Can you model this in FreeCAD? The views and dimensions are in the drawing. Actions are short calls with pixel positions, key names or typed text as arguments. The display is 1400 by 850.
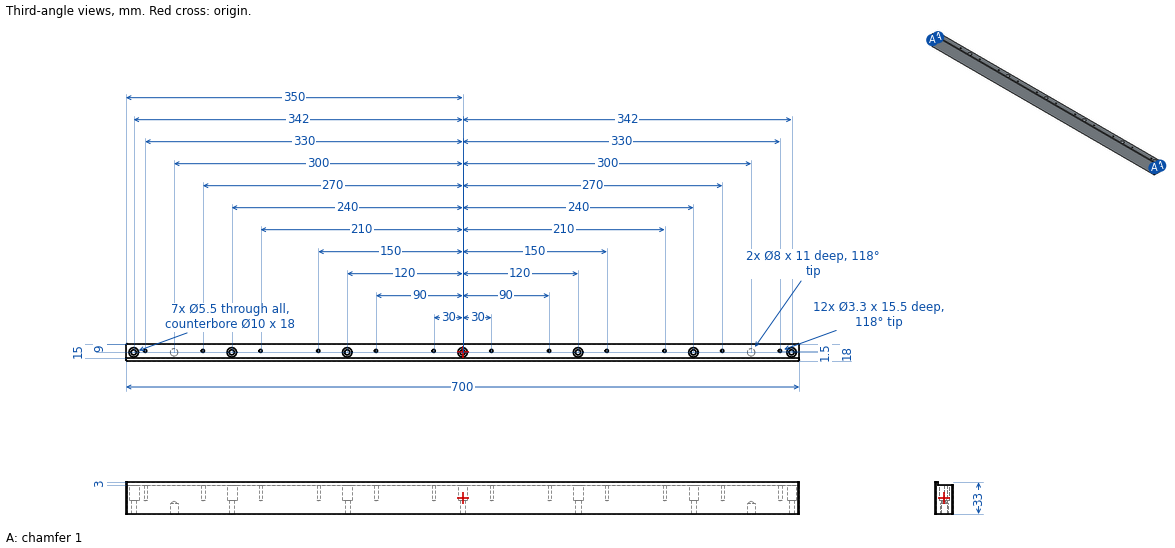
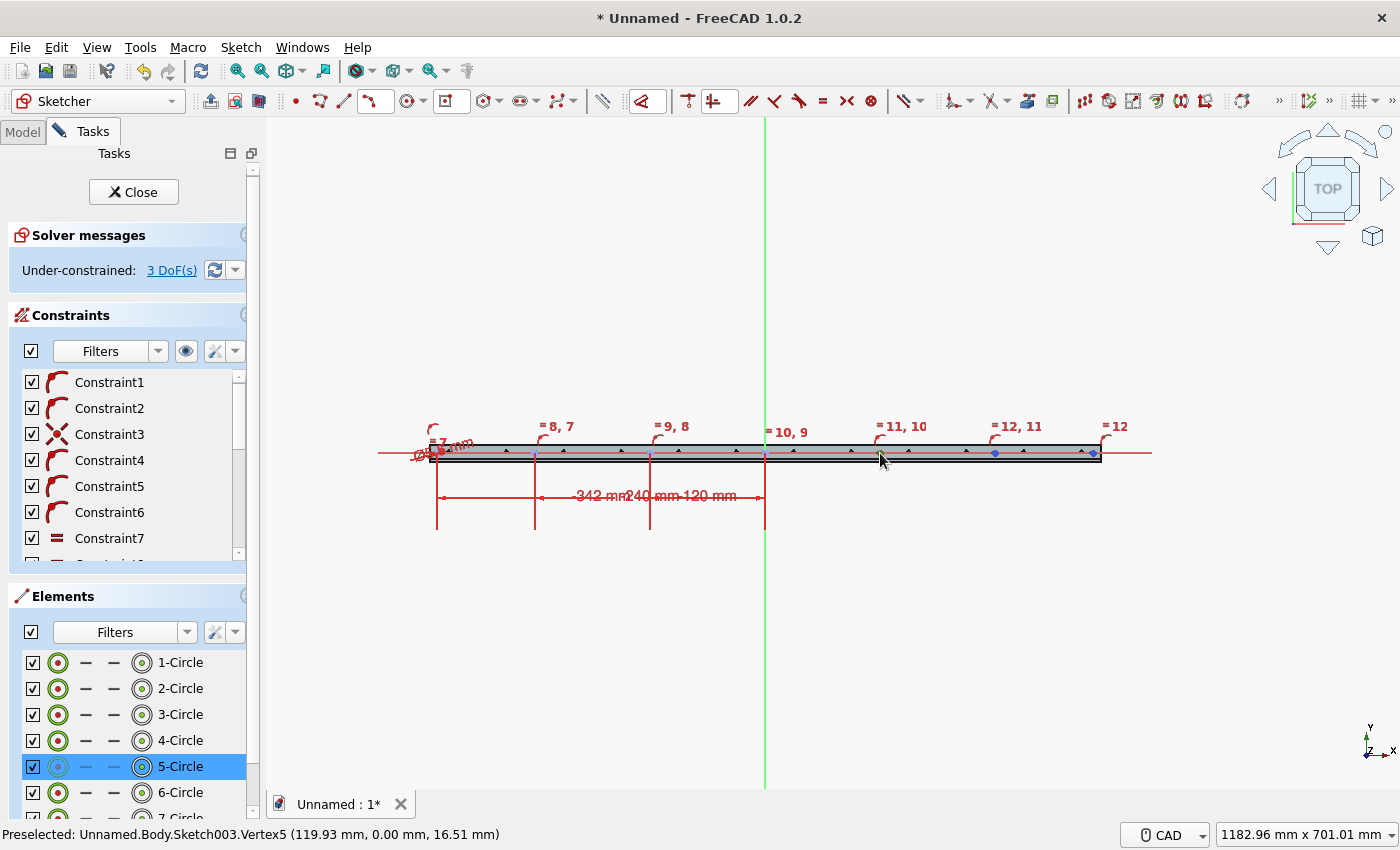
key(l)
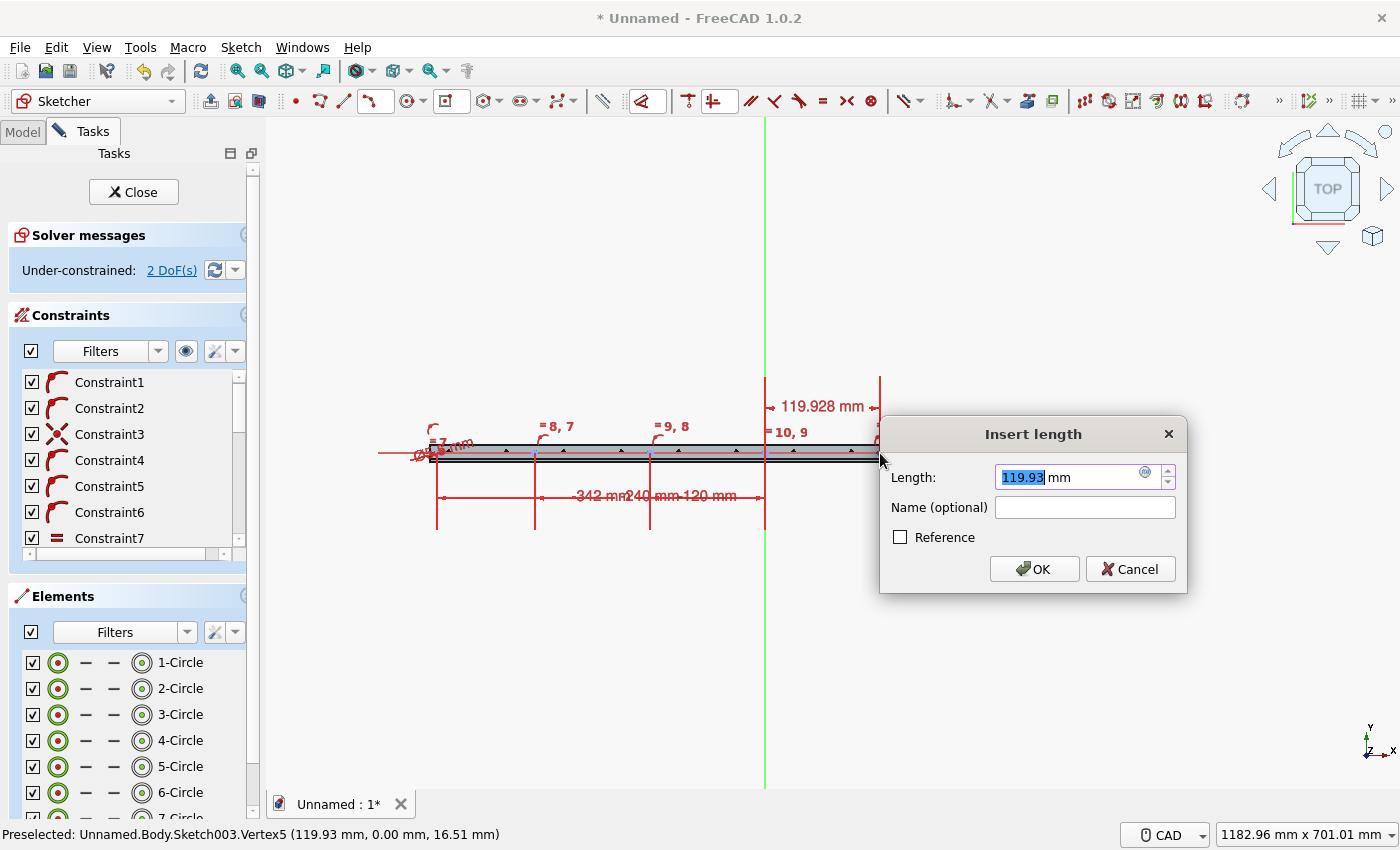
text(120)
key(Return)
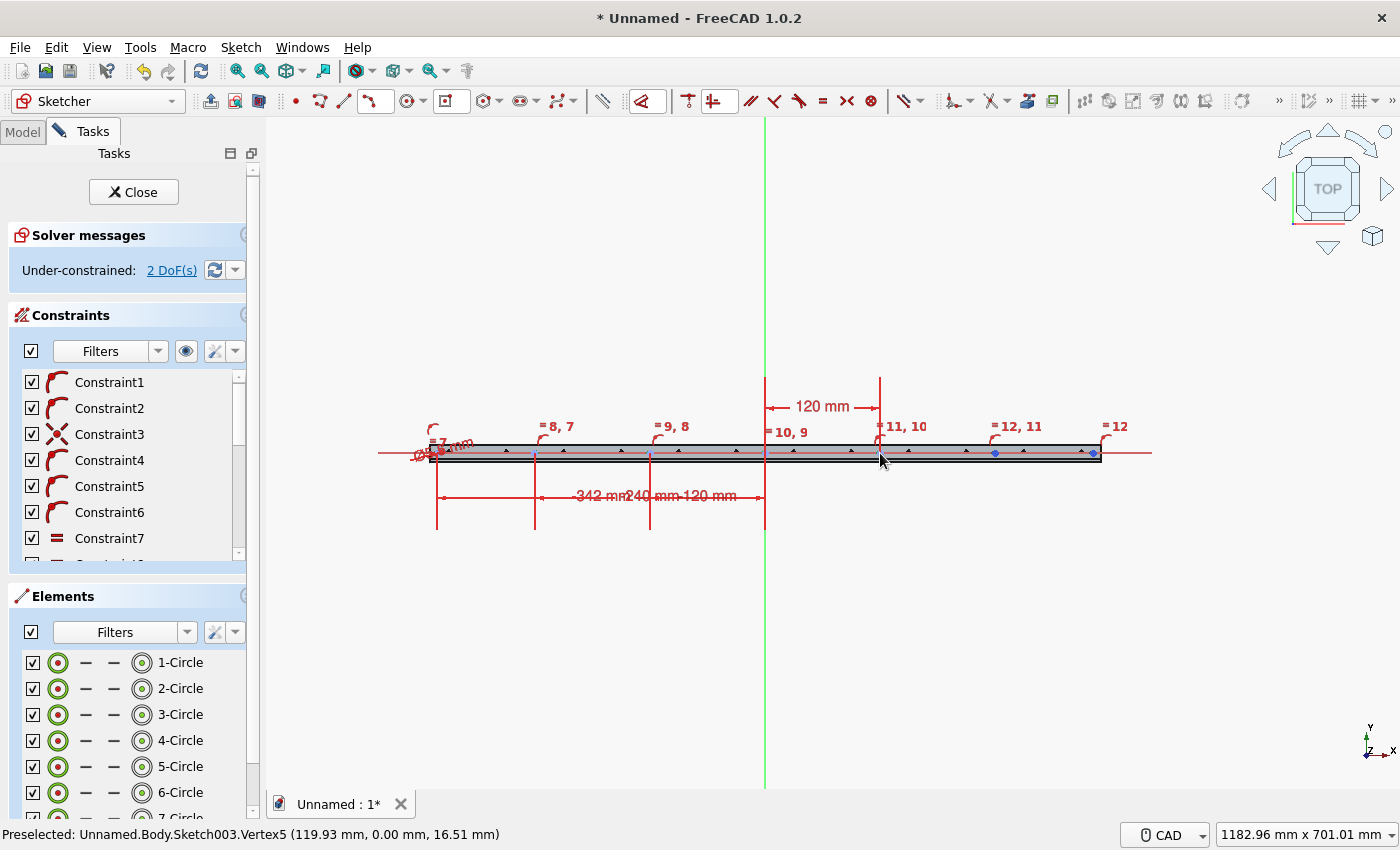
click(995, 453)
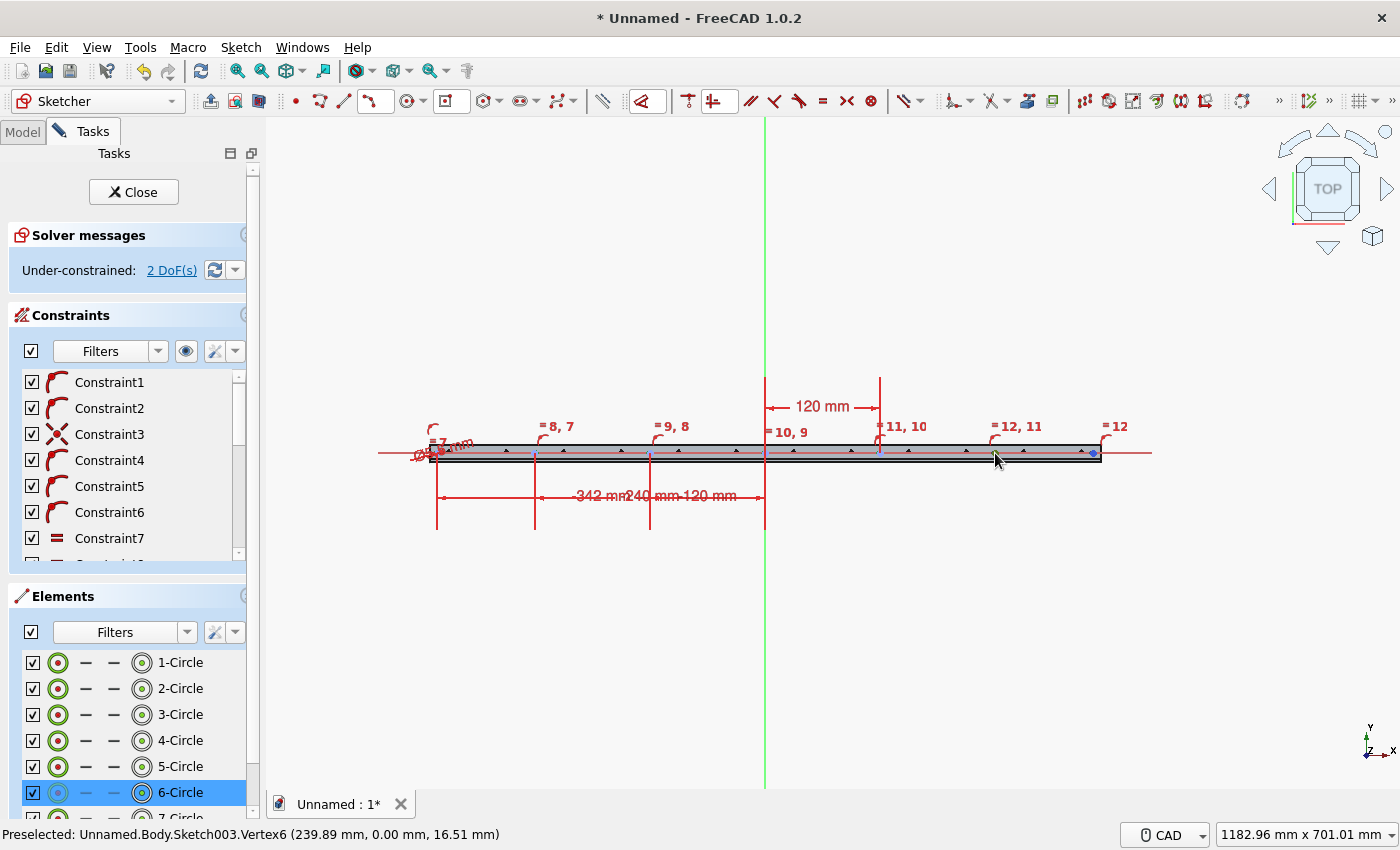
key(l)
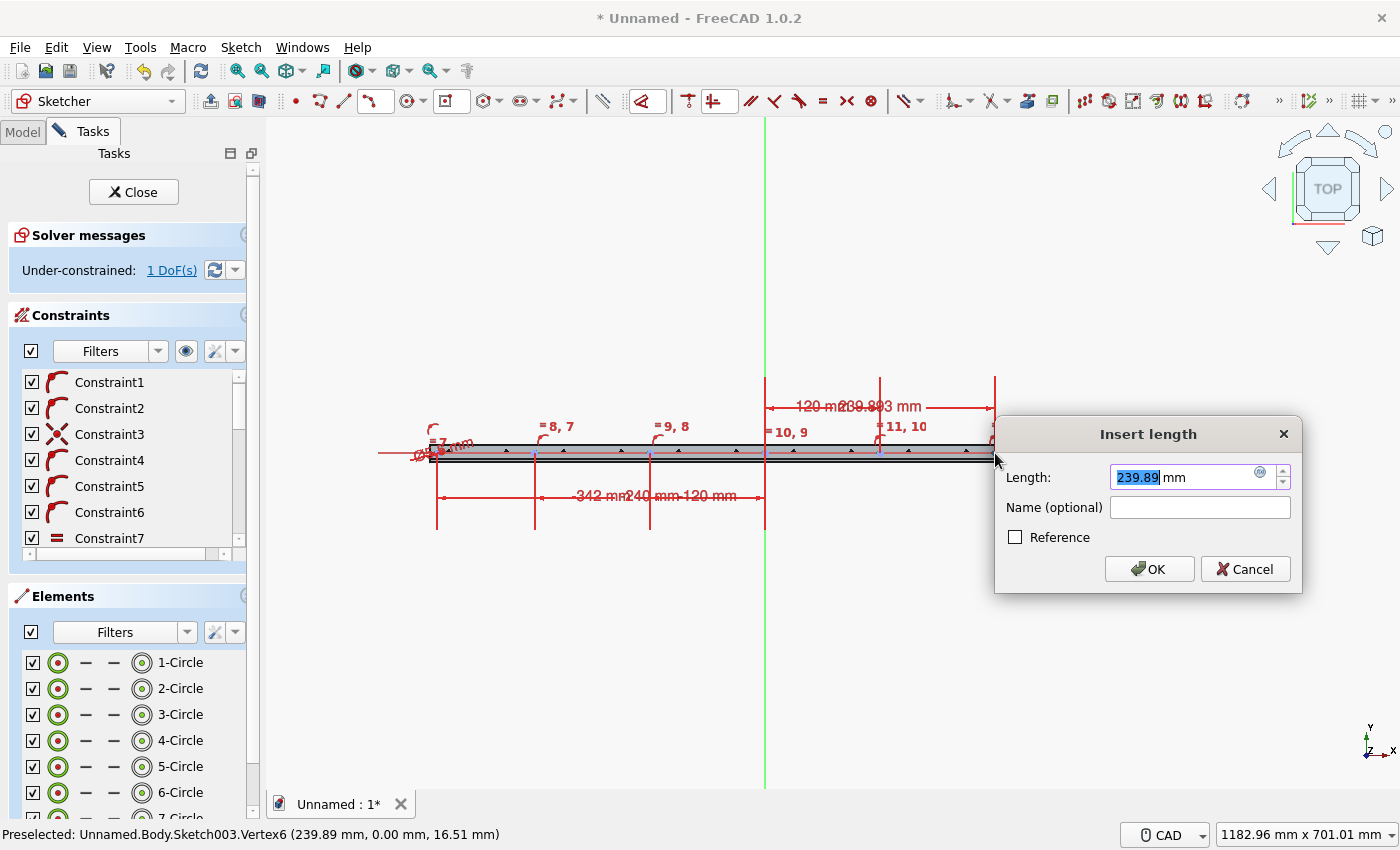
text(240)
key(Return)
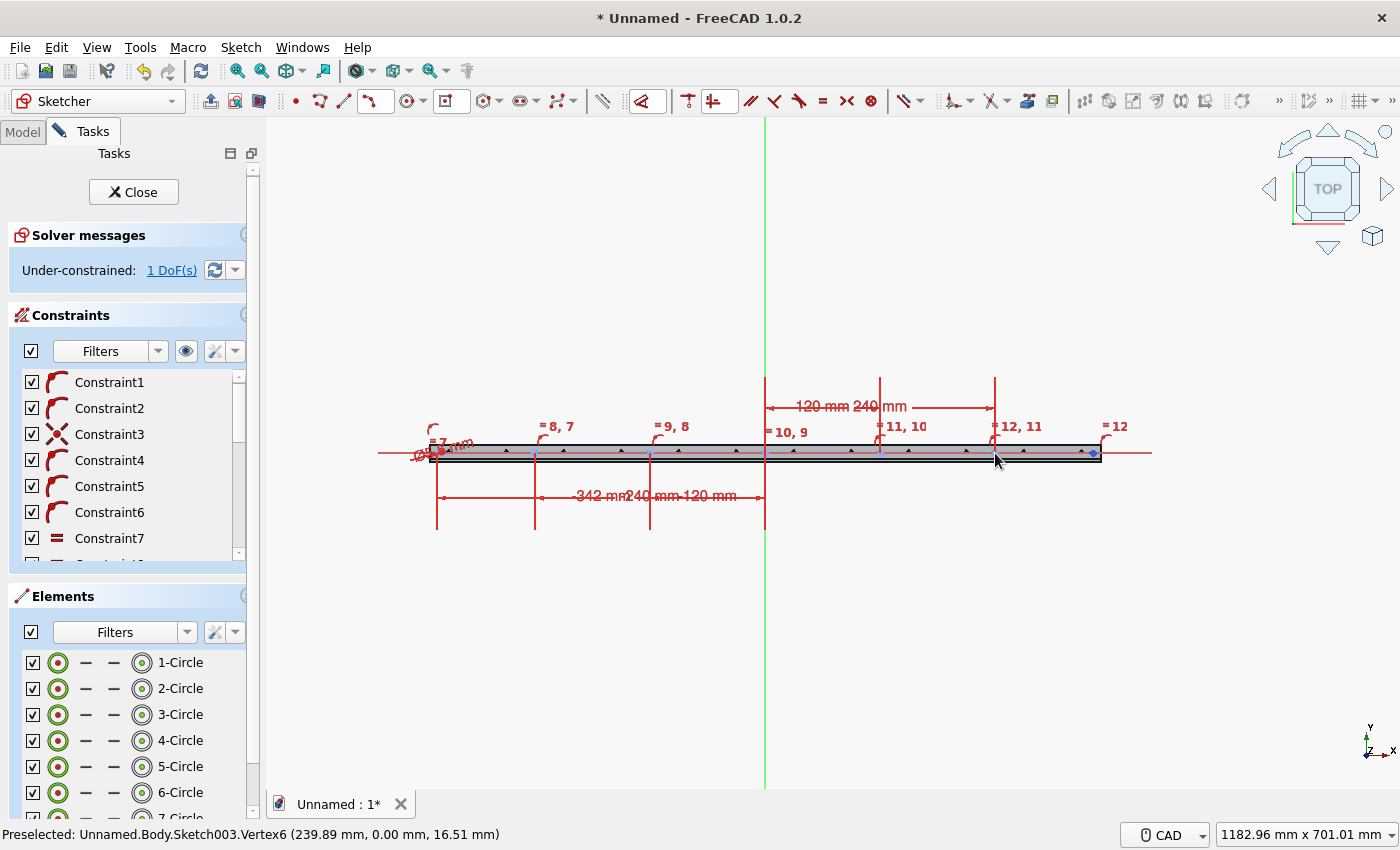
click(1093, 453)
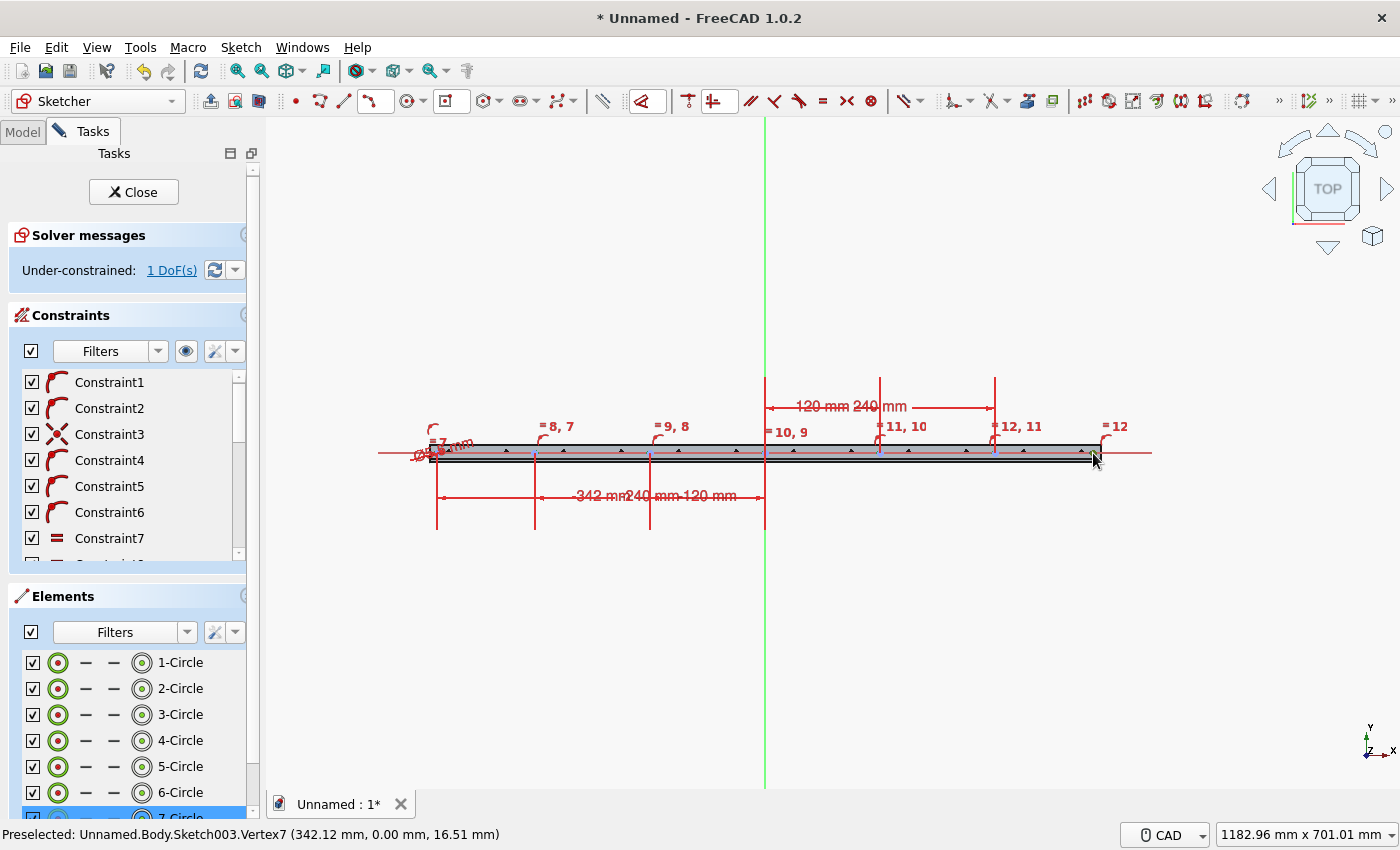
key(l)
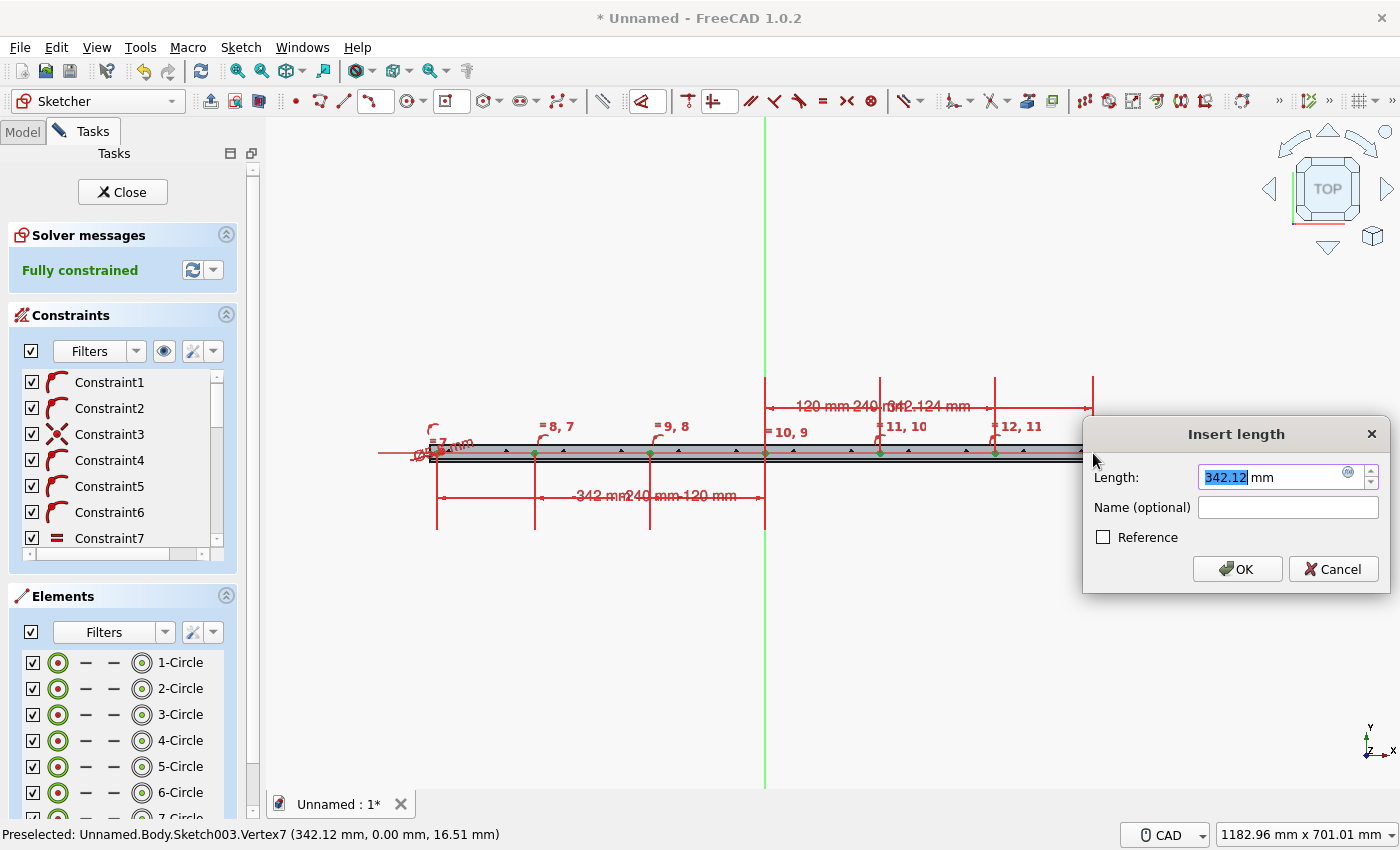
text(342)
key(Return)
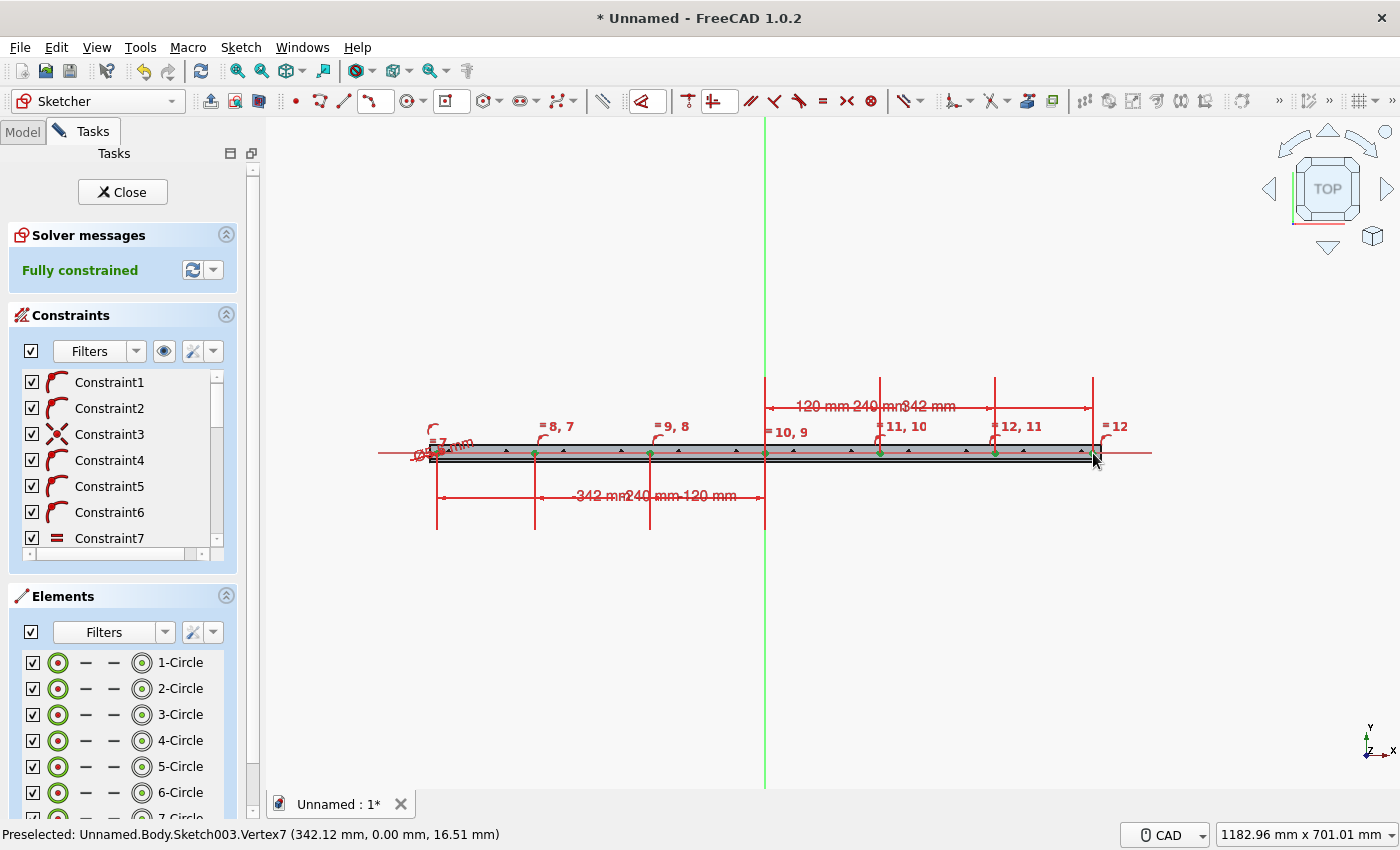
click(123, 192)